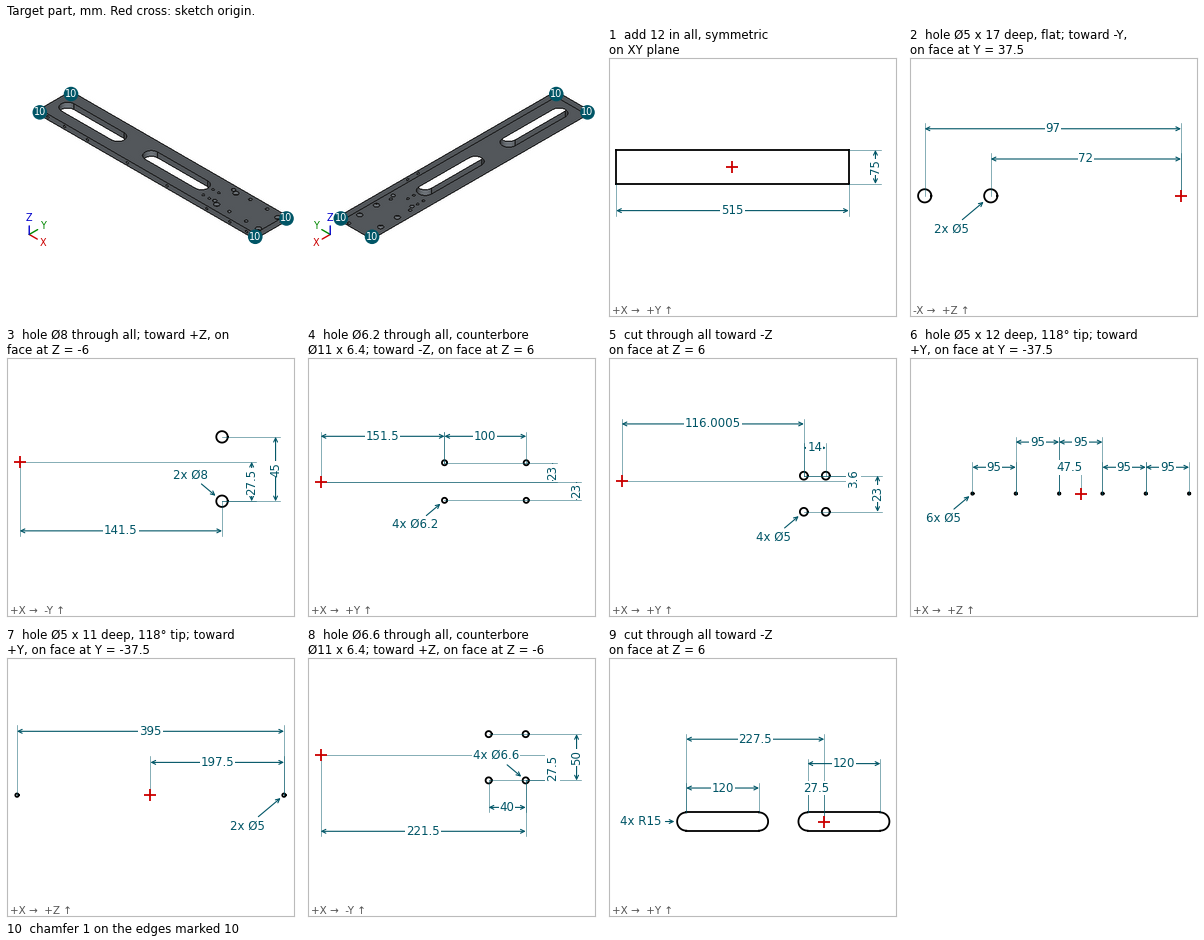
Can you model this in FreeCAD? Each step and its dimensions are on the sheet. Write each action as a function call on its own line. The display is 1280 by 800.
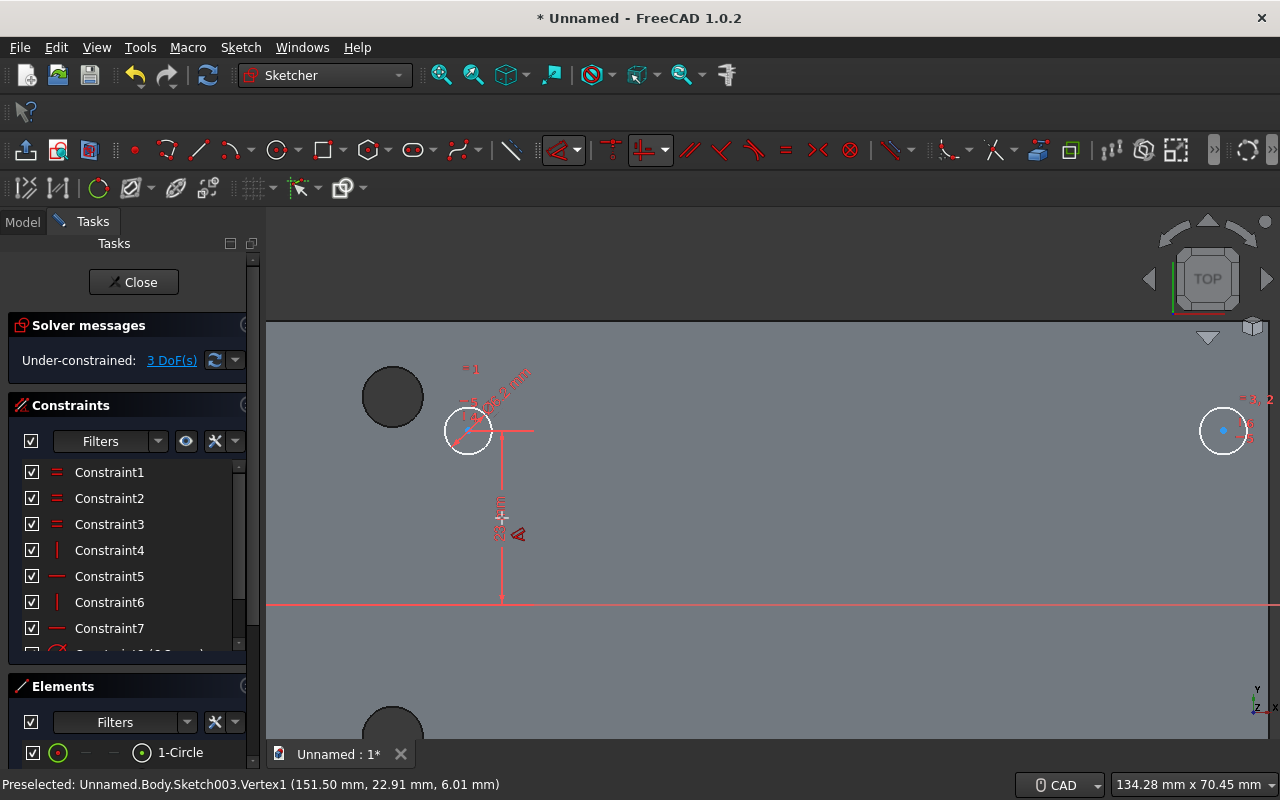
scroll(885, 416, down, 6)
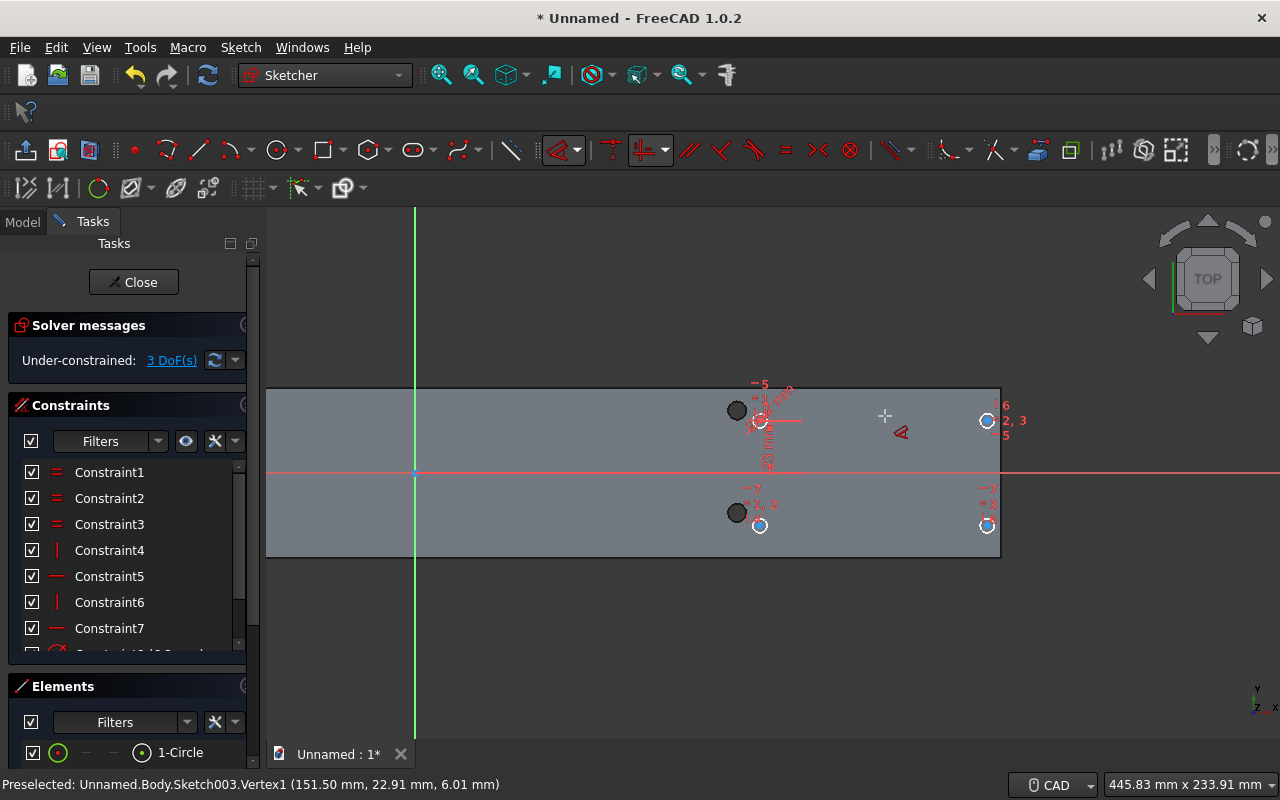
click(760, 526)
click(381, 499)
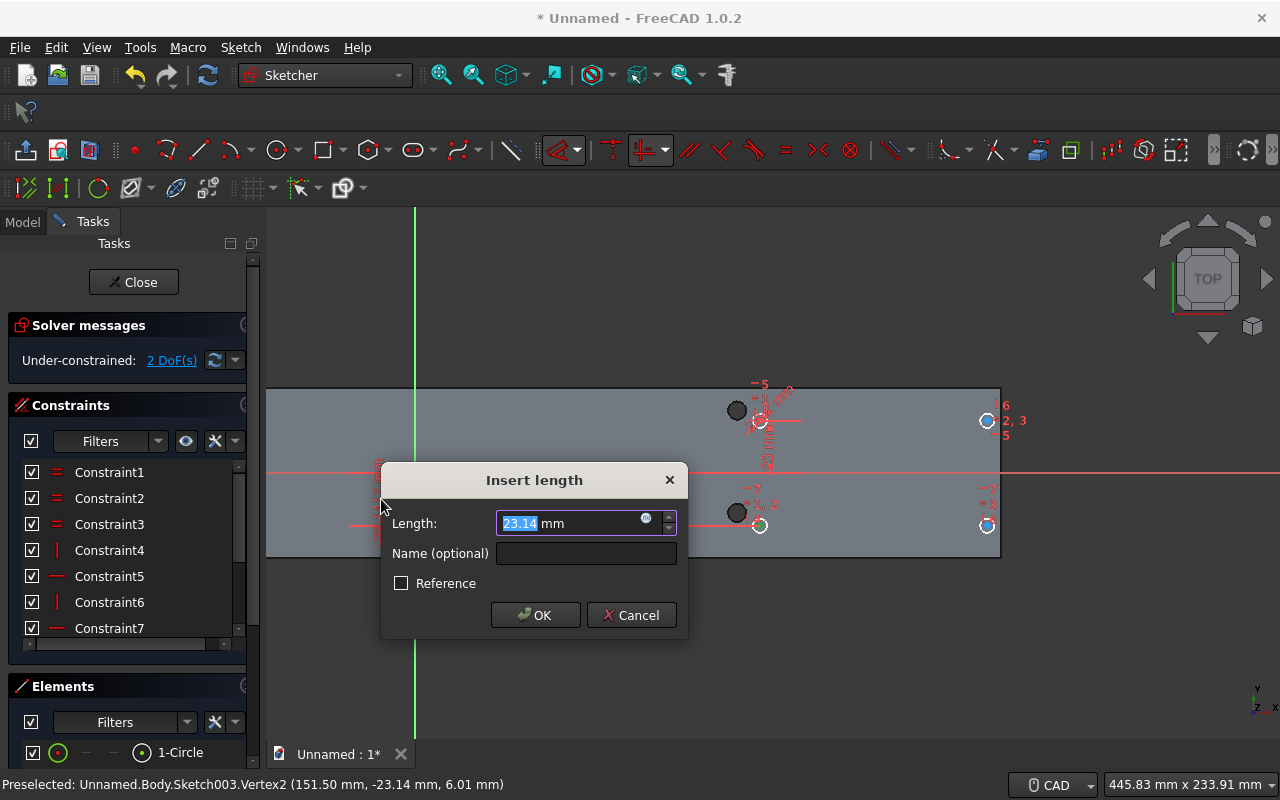
text(23)
key(Return)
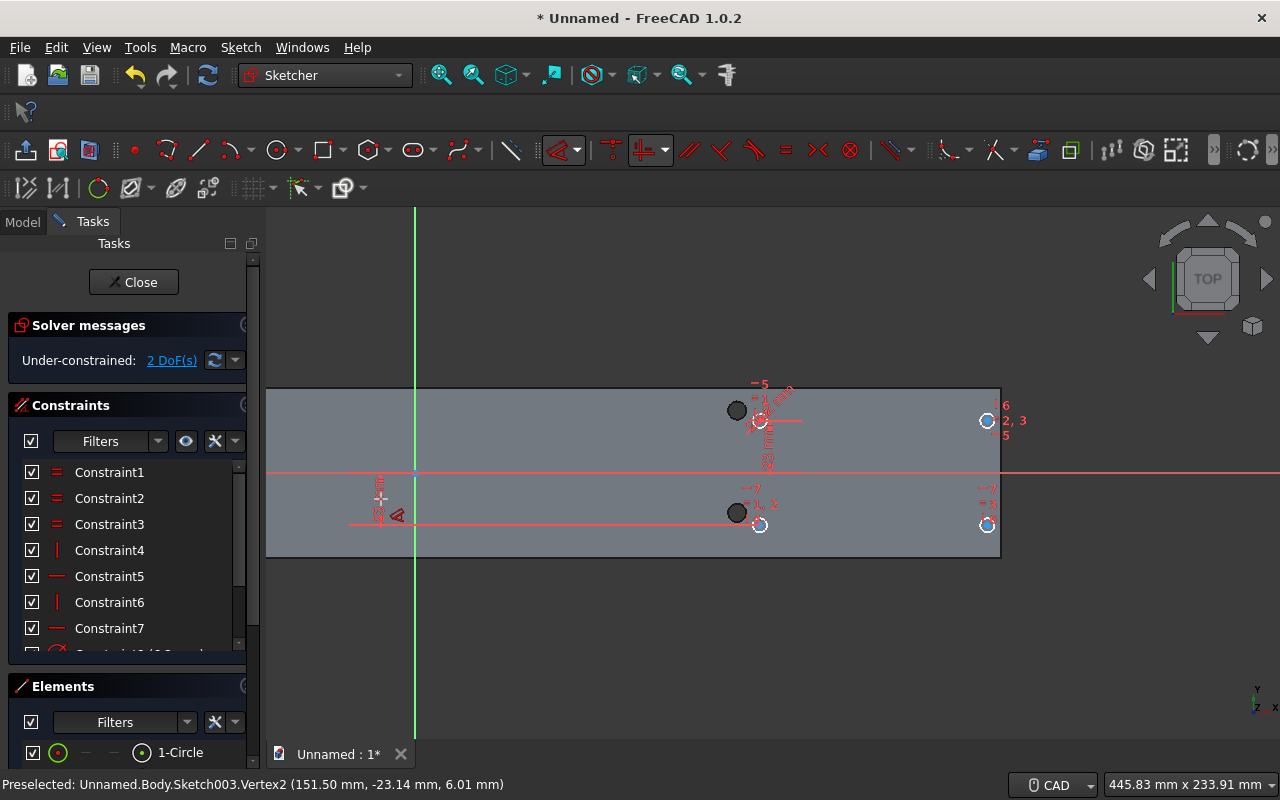
click(760, 421)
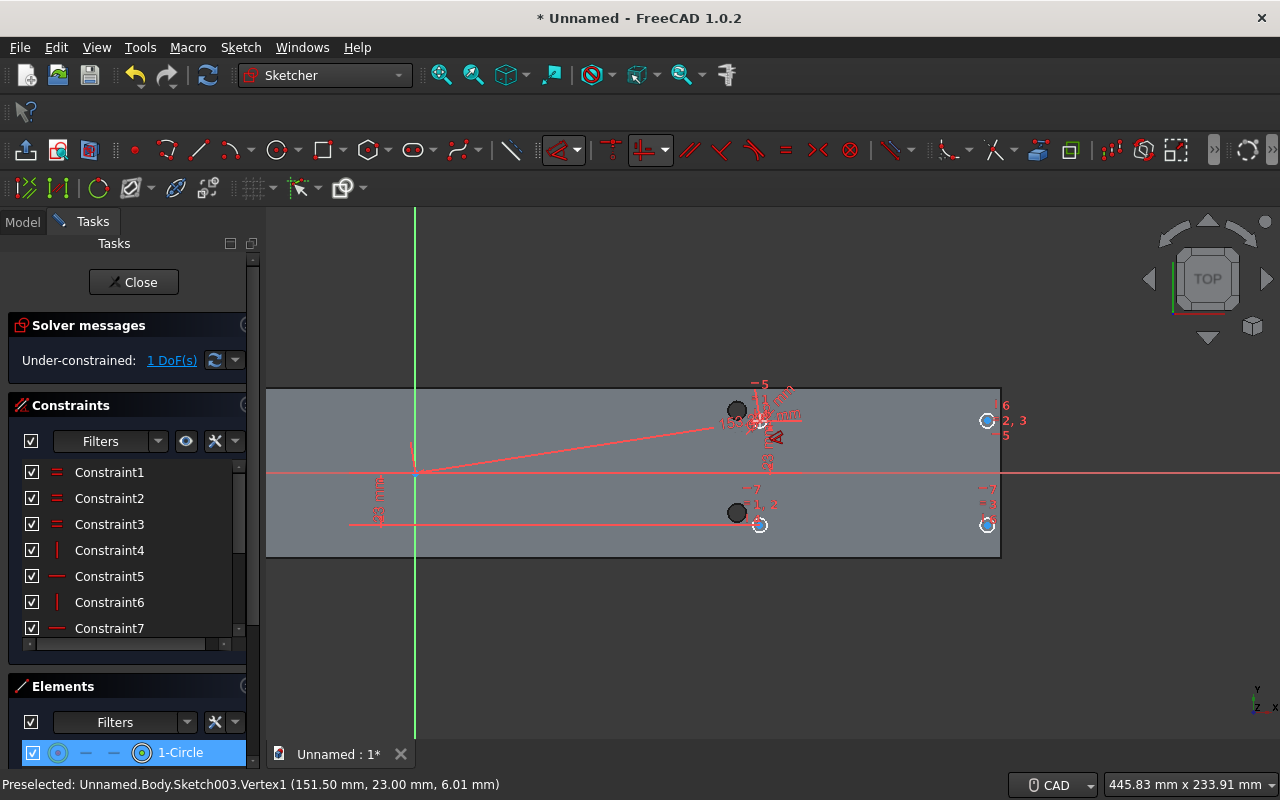
click(987, 421)
click(874, 387)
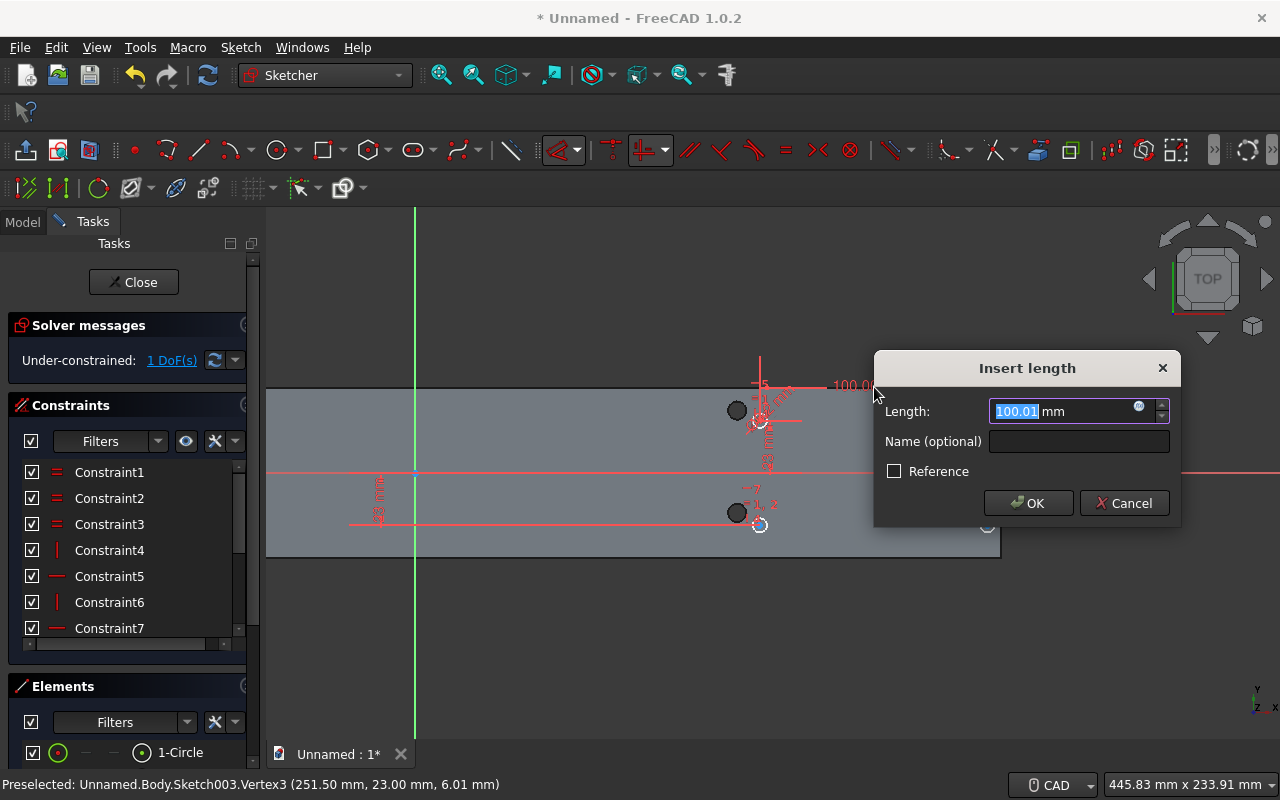
text(100)
key(Return)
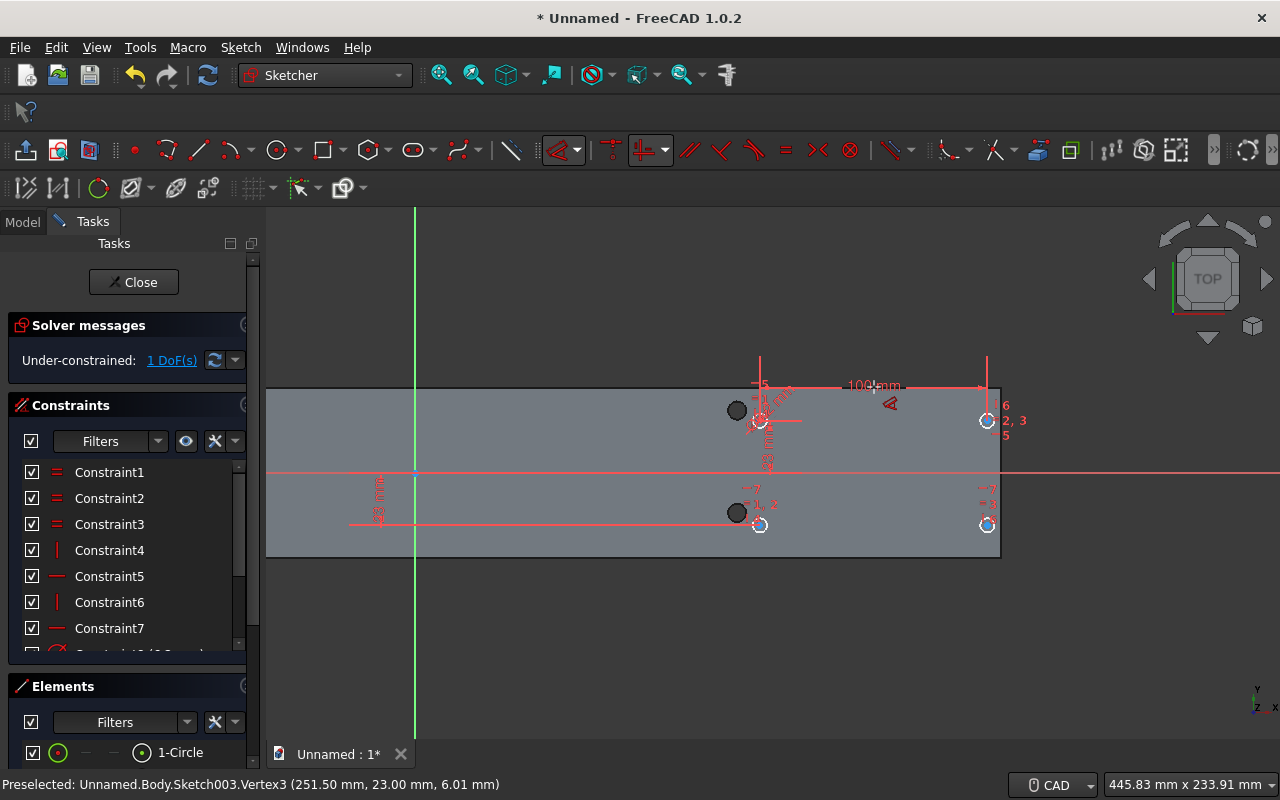
click(760, 421)
click(588, 387)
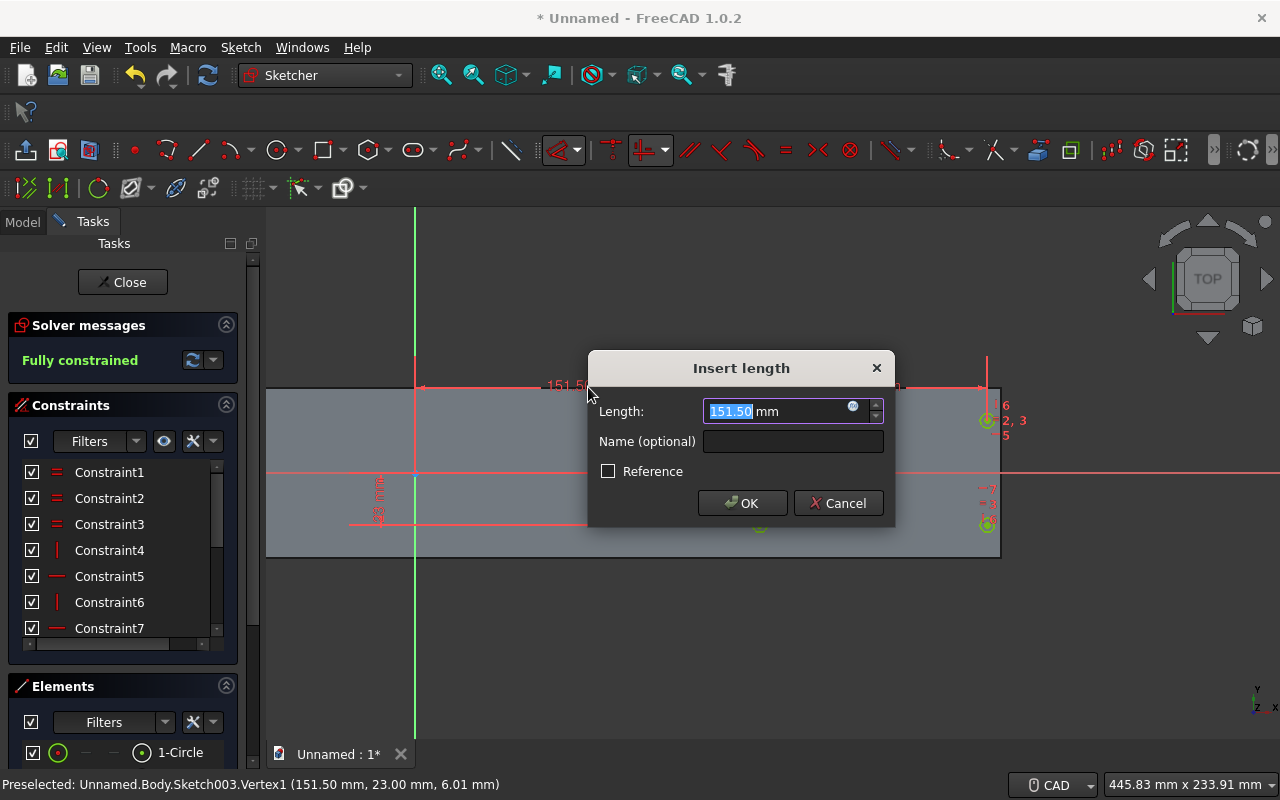
text(151.5)
key(Return)
key(Escape)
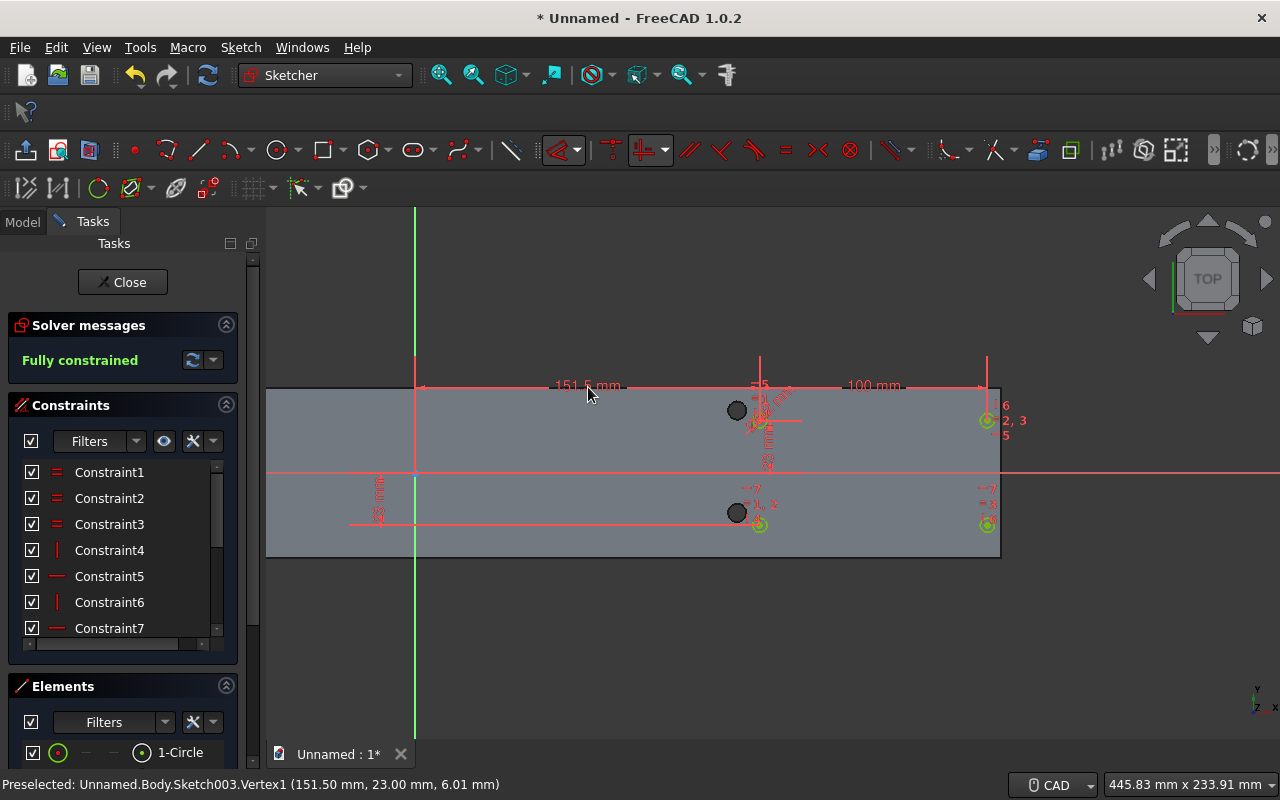
click(123, 282)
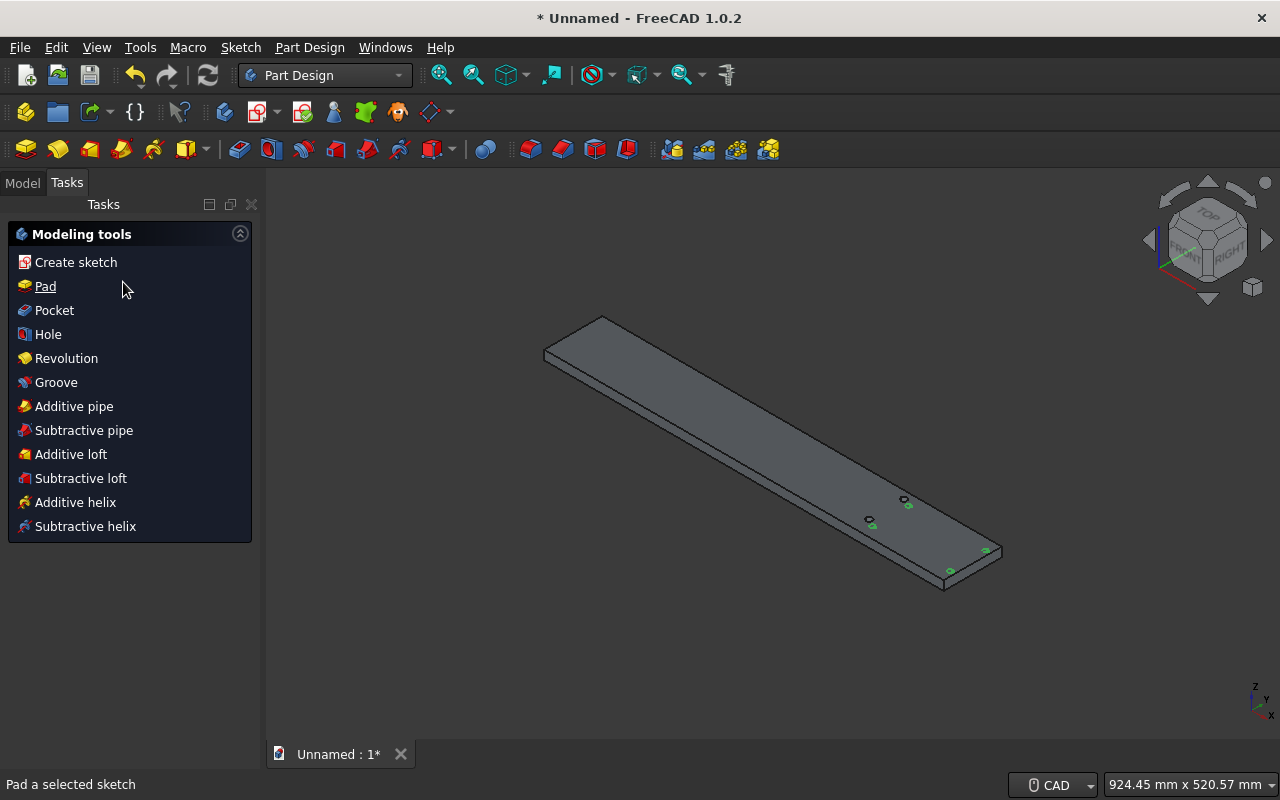
click(272, 150)